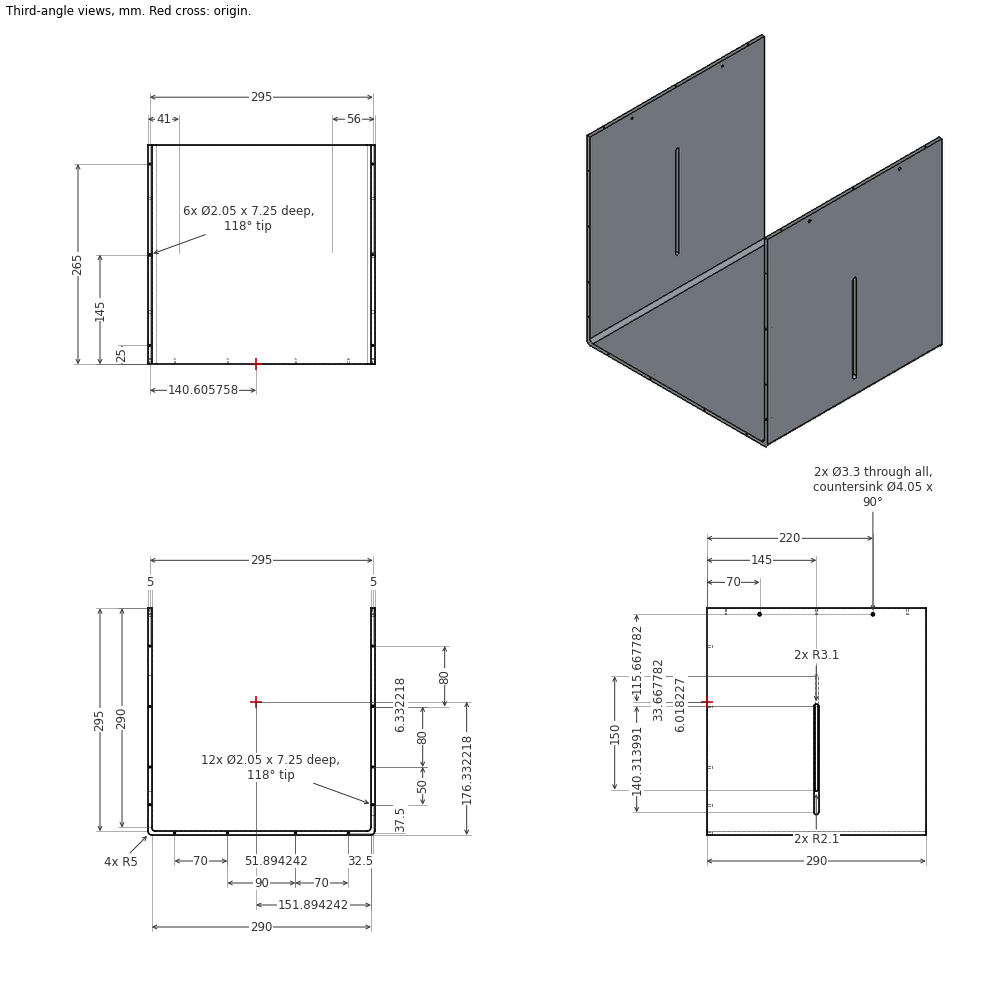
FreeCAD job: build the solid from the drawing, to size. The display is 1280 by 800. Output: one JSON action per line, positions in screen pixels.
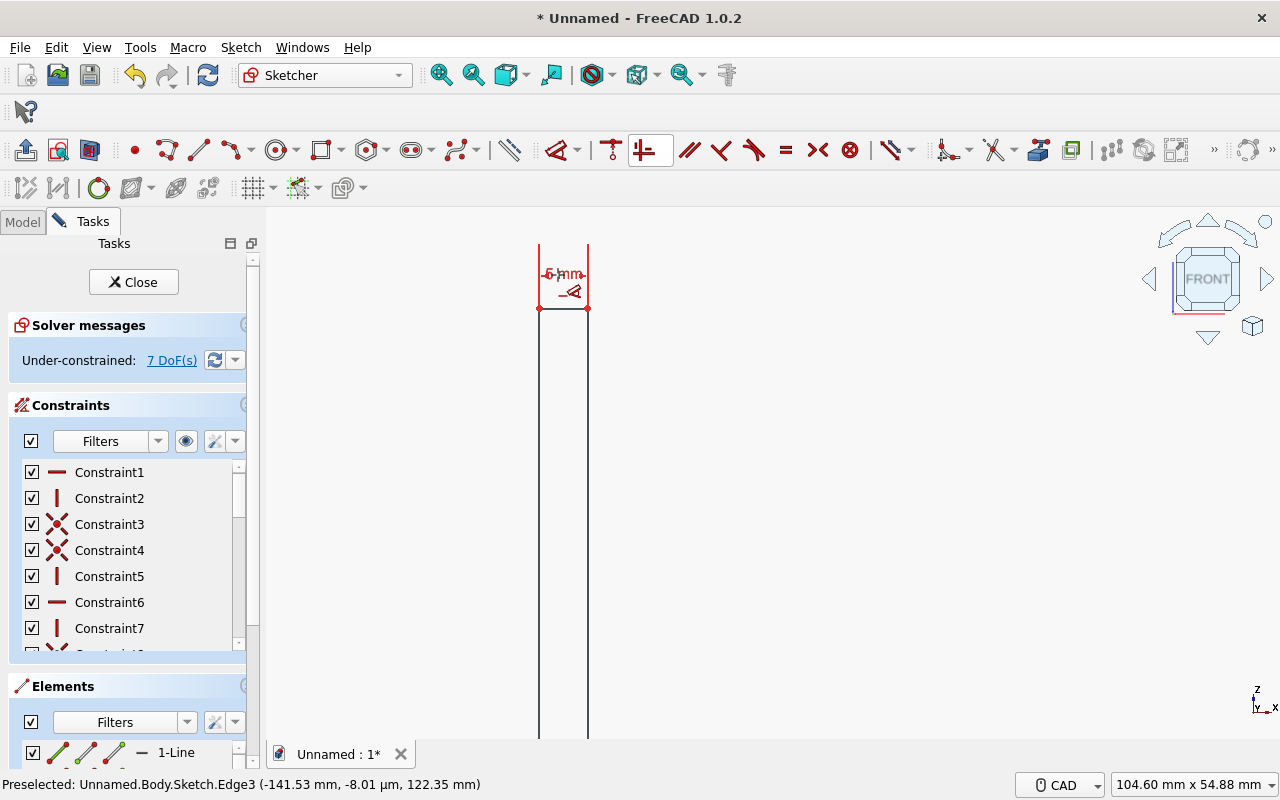
{"action": "scroll", "coordinate": [545, 314], "scroll_direction": "down", "scroll_amount": 11}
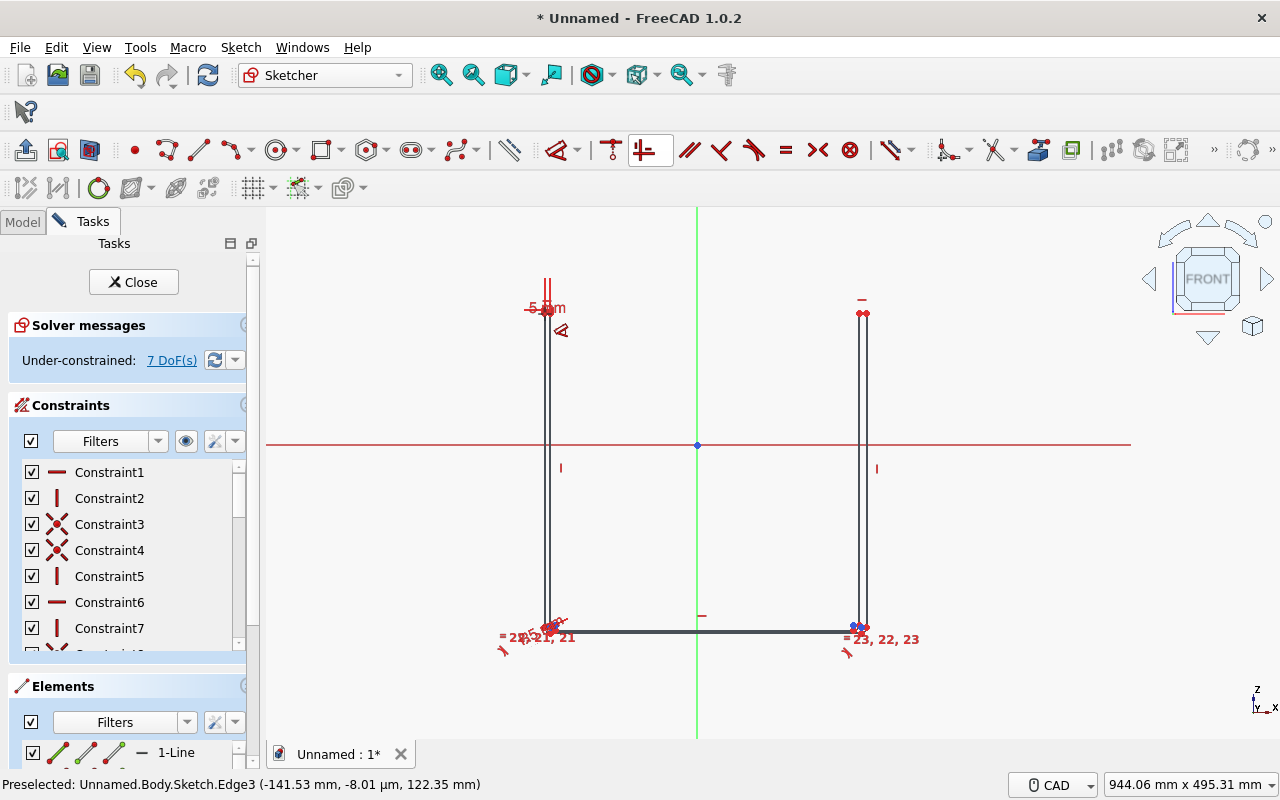
{"action": "scroll", "coordinate": [861, 313], "scroll_direction": "up", "scroll_amount": 11}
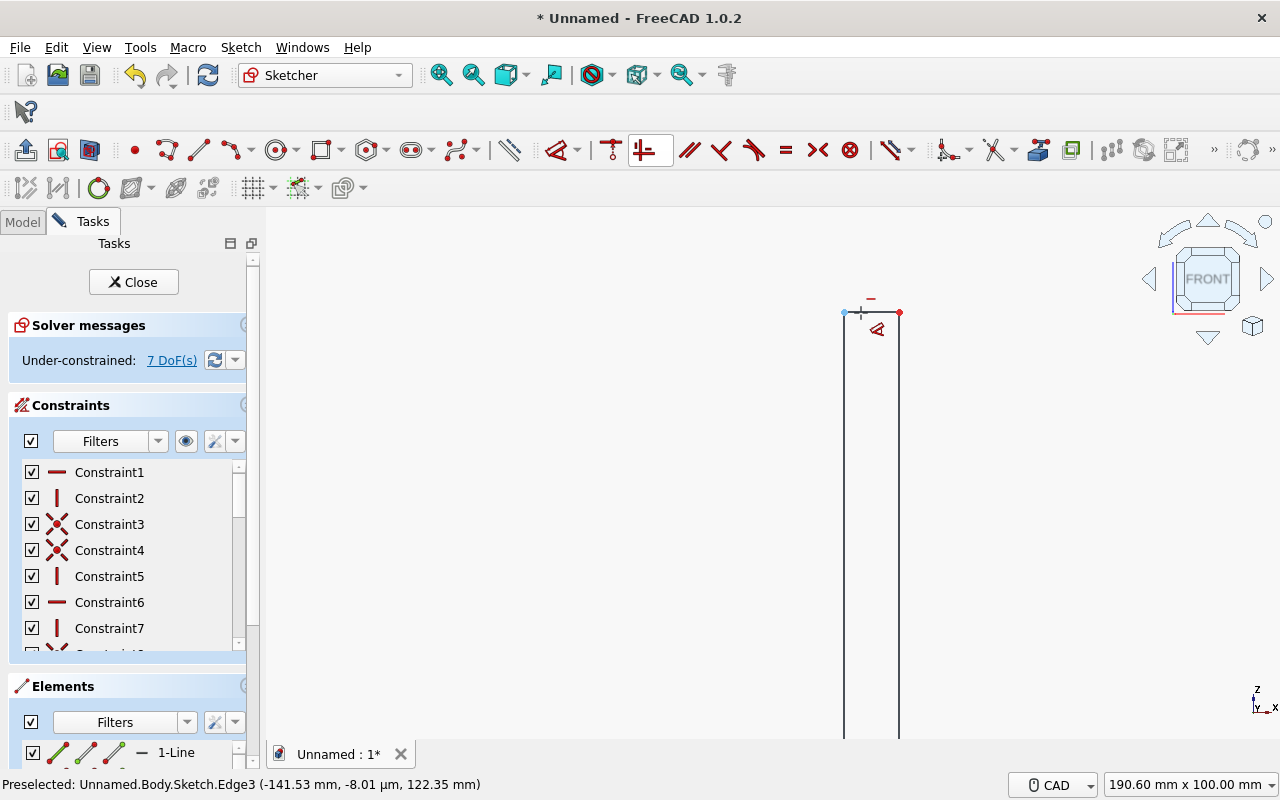
{"action": "left_click", "coordinate": [861, 312]}
{"action": "left_click", "coordinate": [874, 278]}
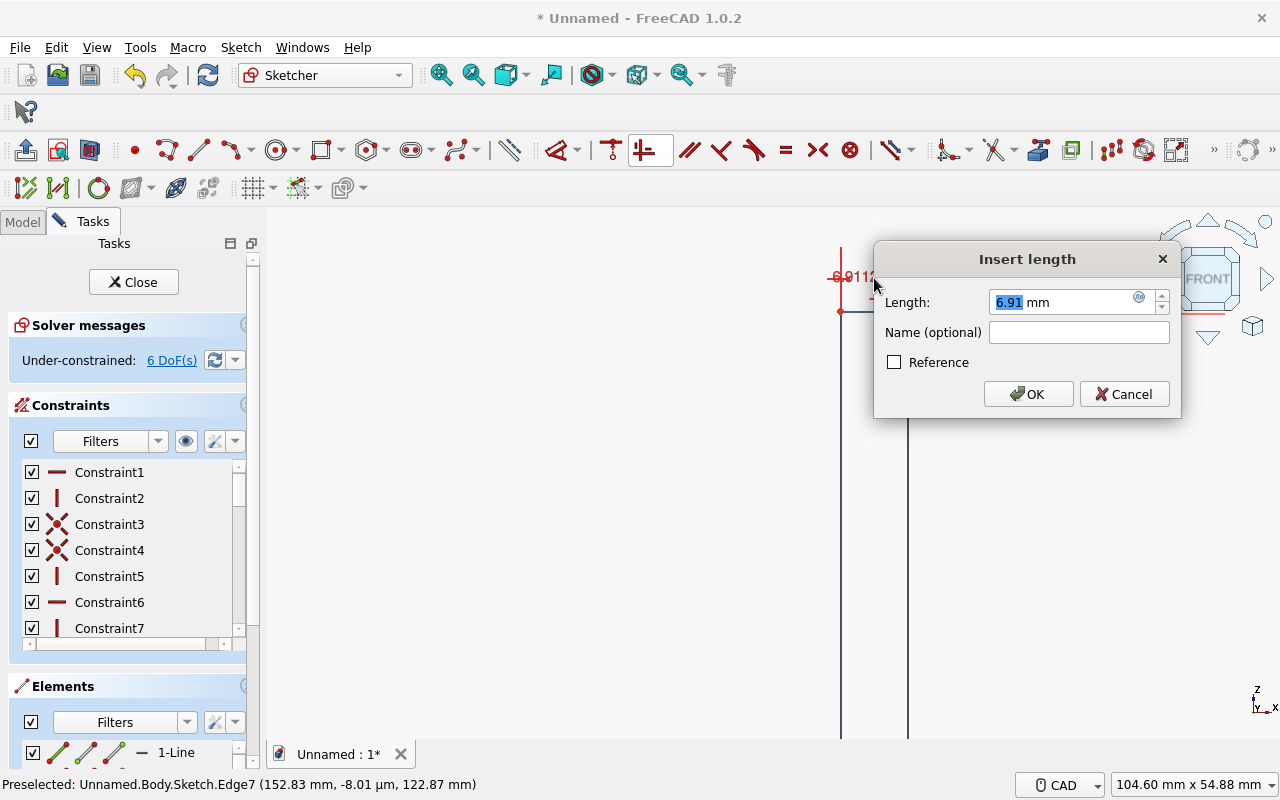
{"action": "type", "text": "5"}
{"action": "key", "text": "Return"}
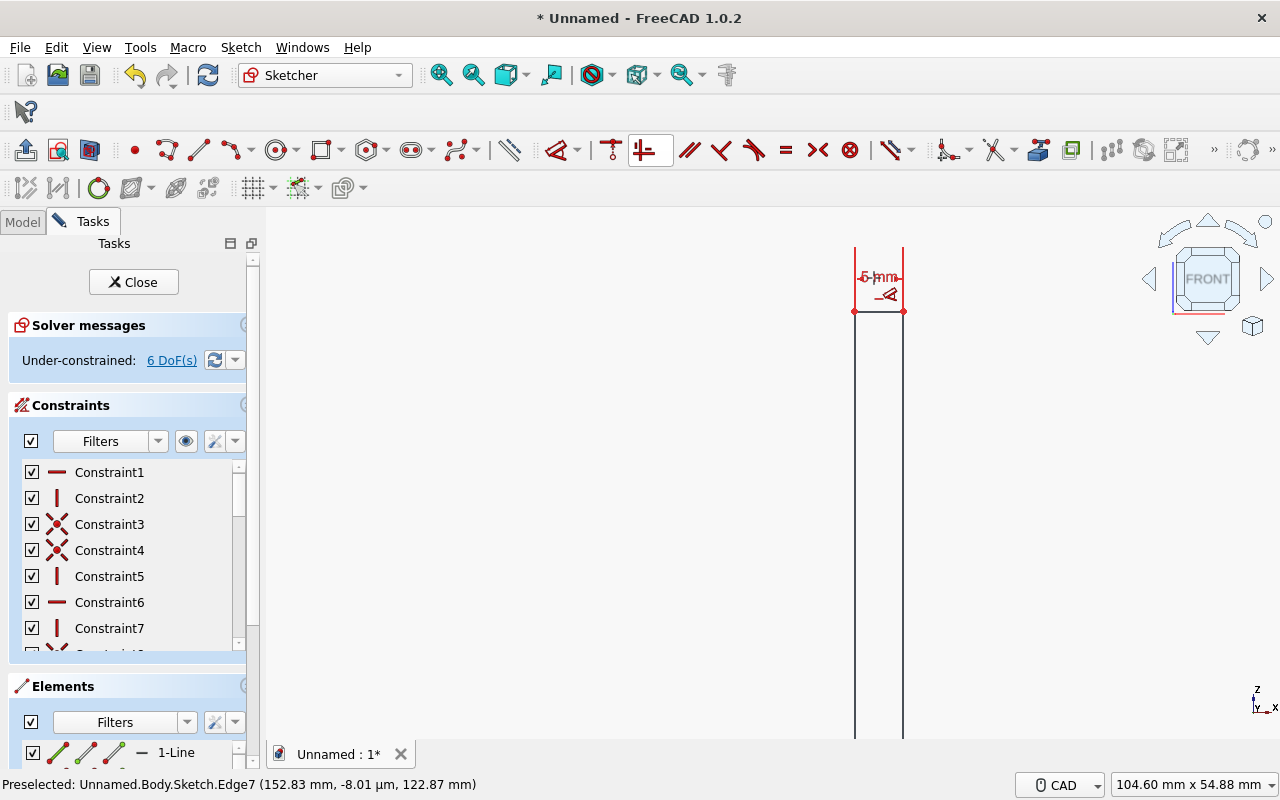
{"action": "scroll", "coordinate": [861, 313], "scroll_direction": "down", "scroll_amount": 11}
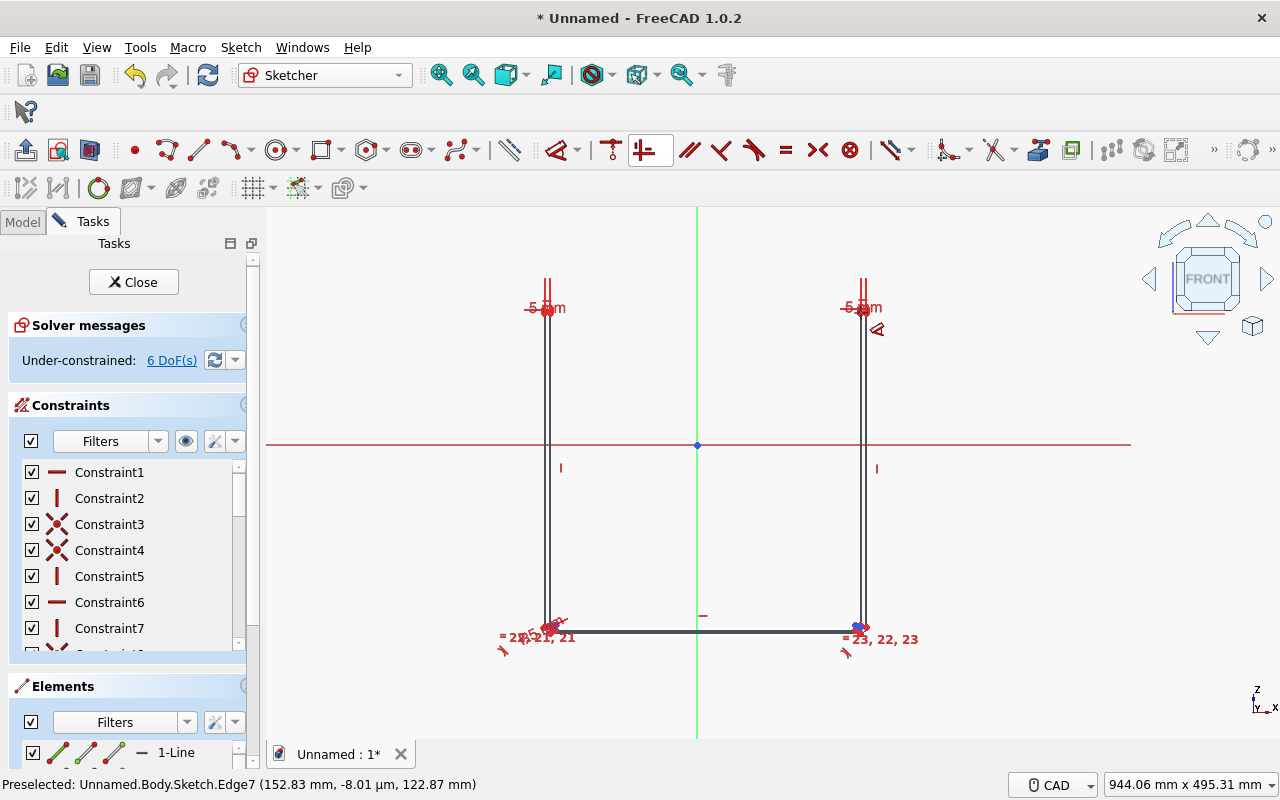
{"action": "scroll", "coordinate": [768, 633], "scroll_direction": "up", "scroll_amount": 9}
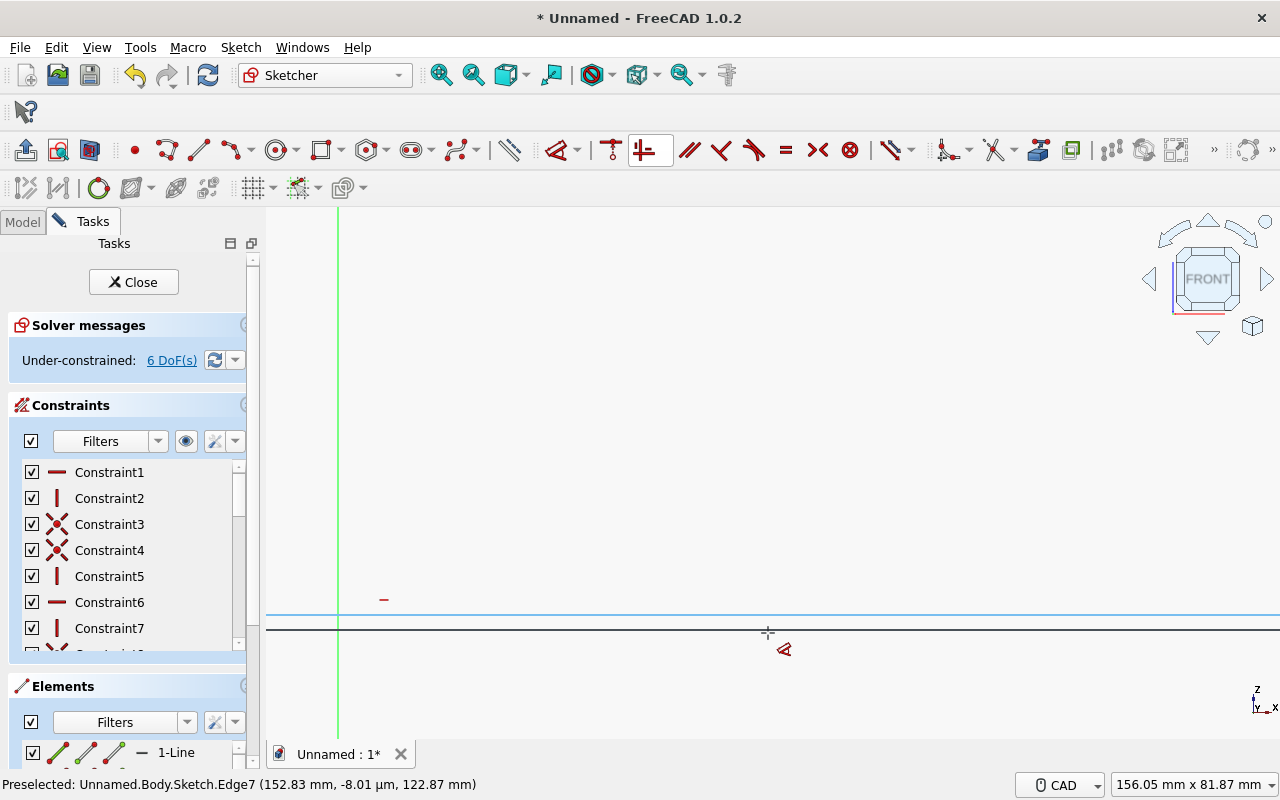
{"action": "left_click", "coordinate": [763, 630]}
{"action": "left_click", "coordinate": [704, 664]}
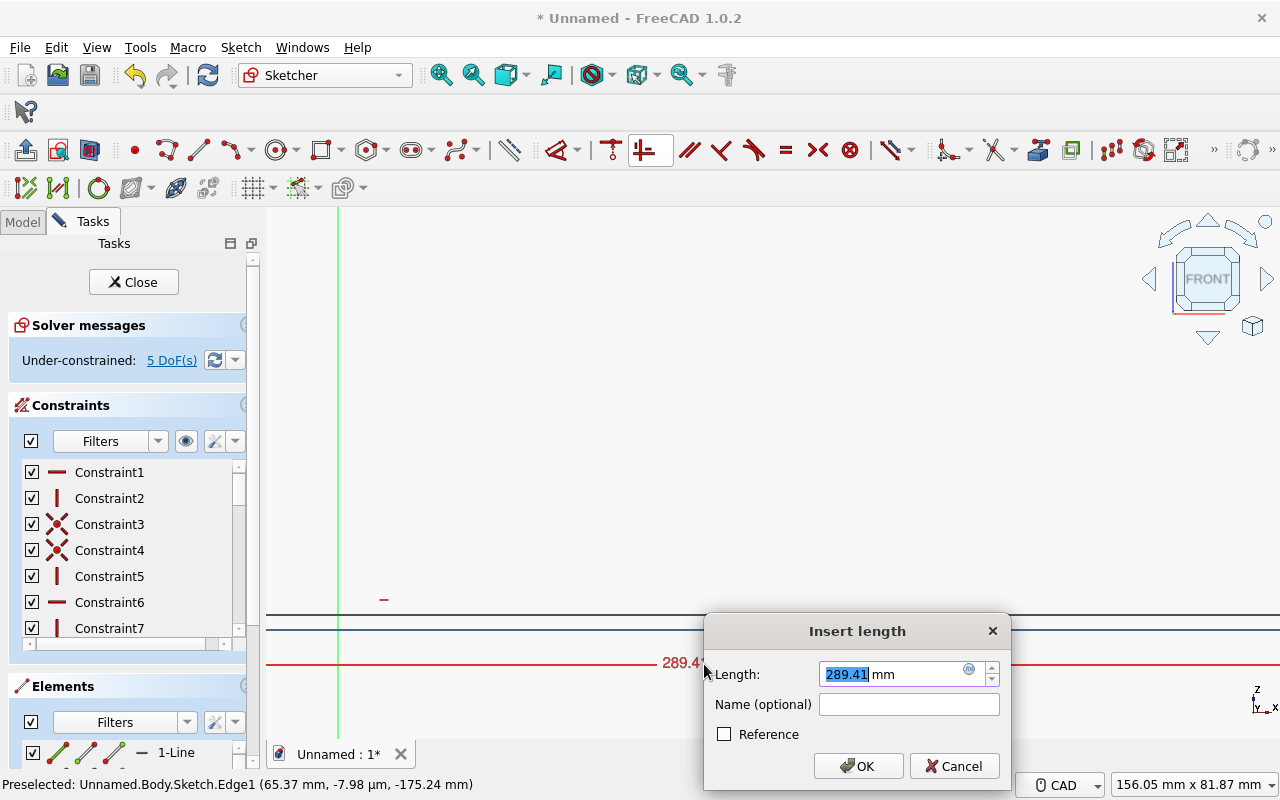
{"action": "type", "text": "290"}
{"action": "key", "text": "Return"}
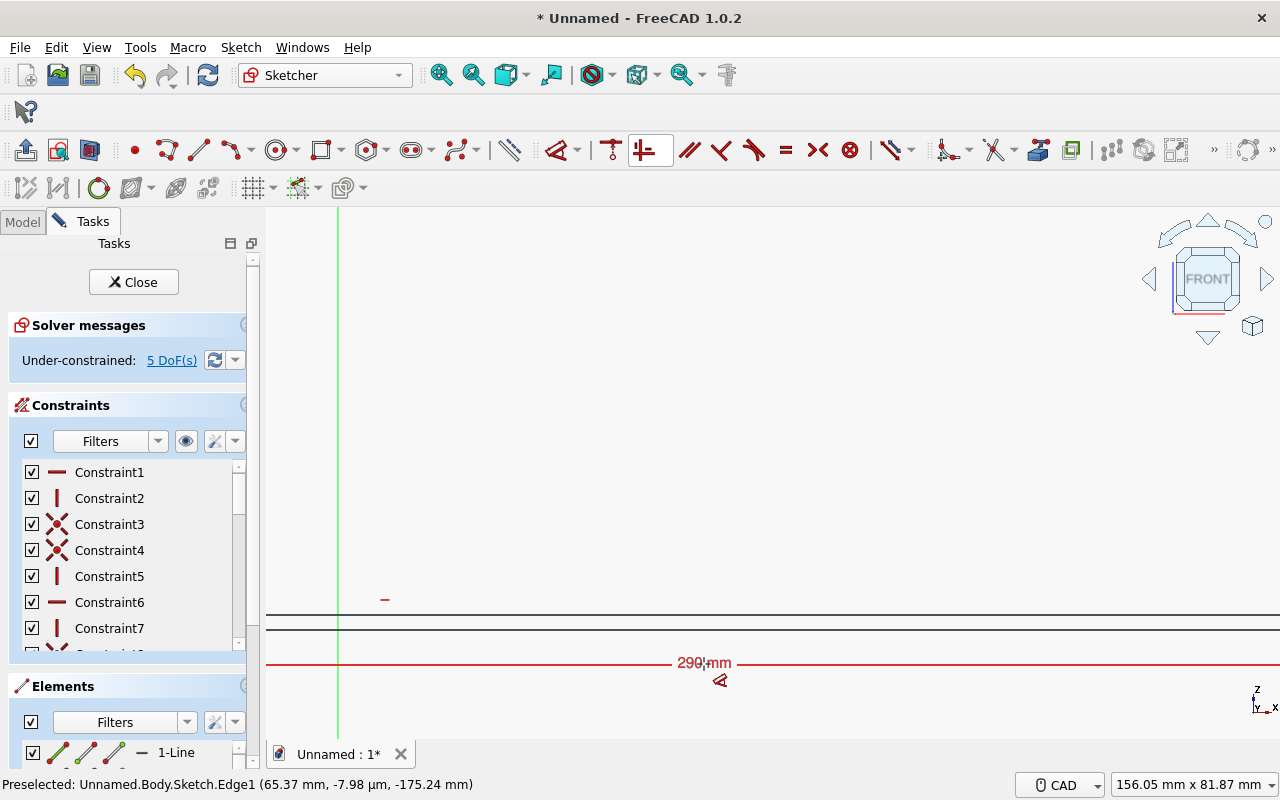
{"action": "scroll", "coordinate": [768, 633], "scroll_direction": "down", "scroll_amount": 9}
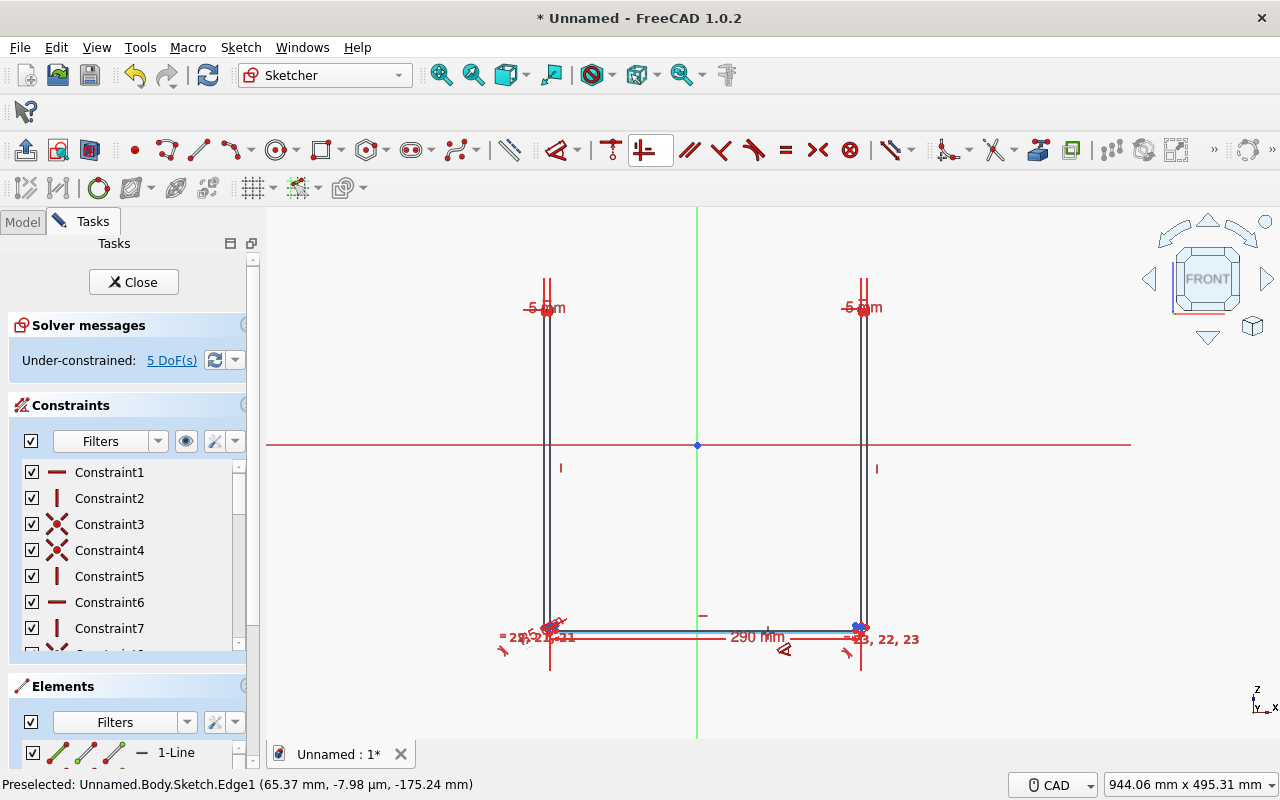
{"action": "scroll", "coordinate": [544, 534], "scroll_direction": "up", "scroll_amount": 5}